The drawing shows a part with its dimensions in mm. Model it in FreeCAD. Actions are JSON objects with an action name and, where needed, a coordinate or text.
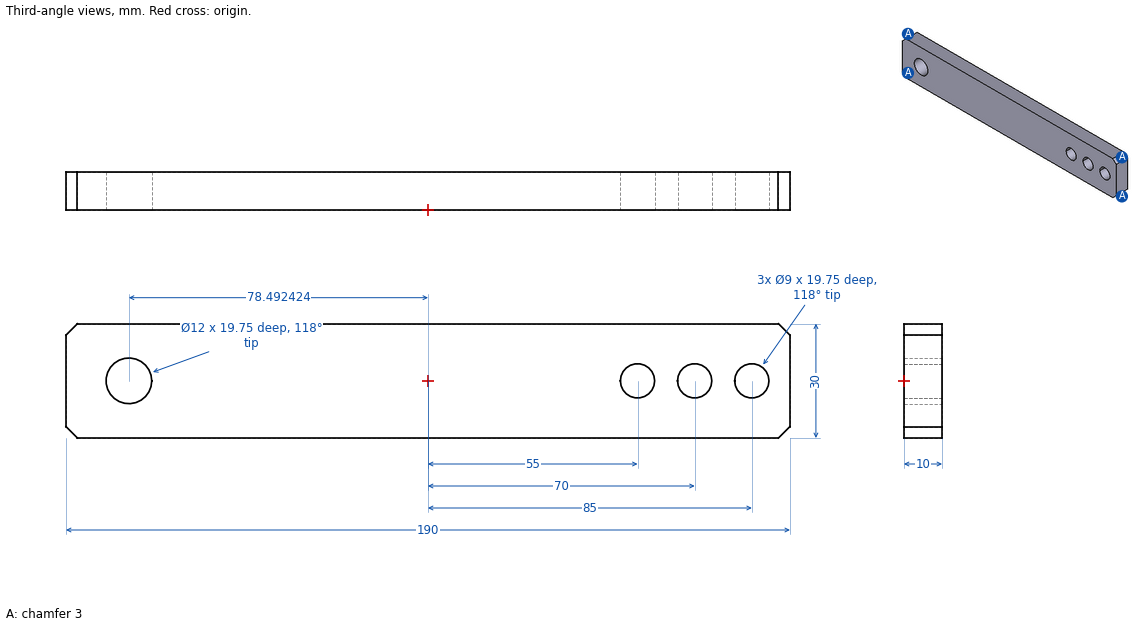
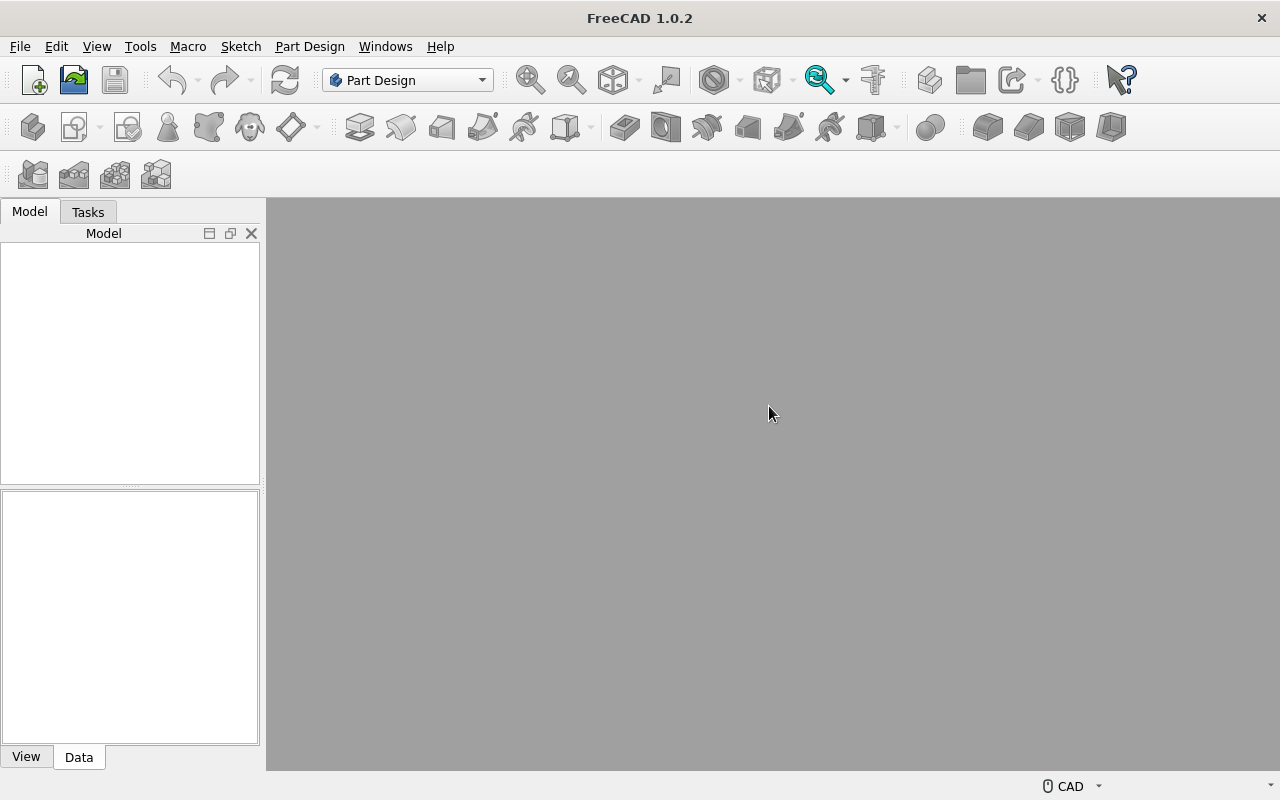
{"action": "key", "text": "ctrl+n"}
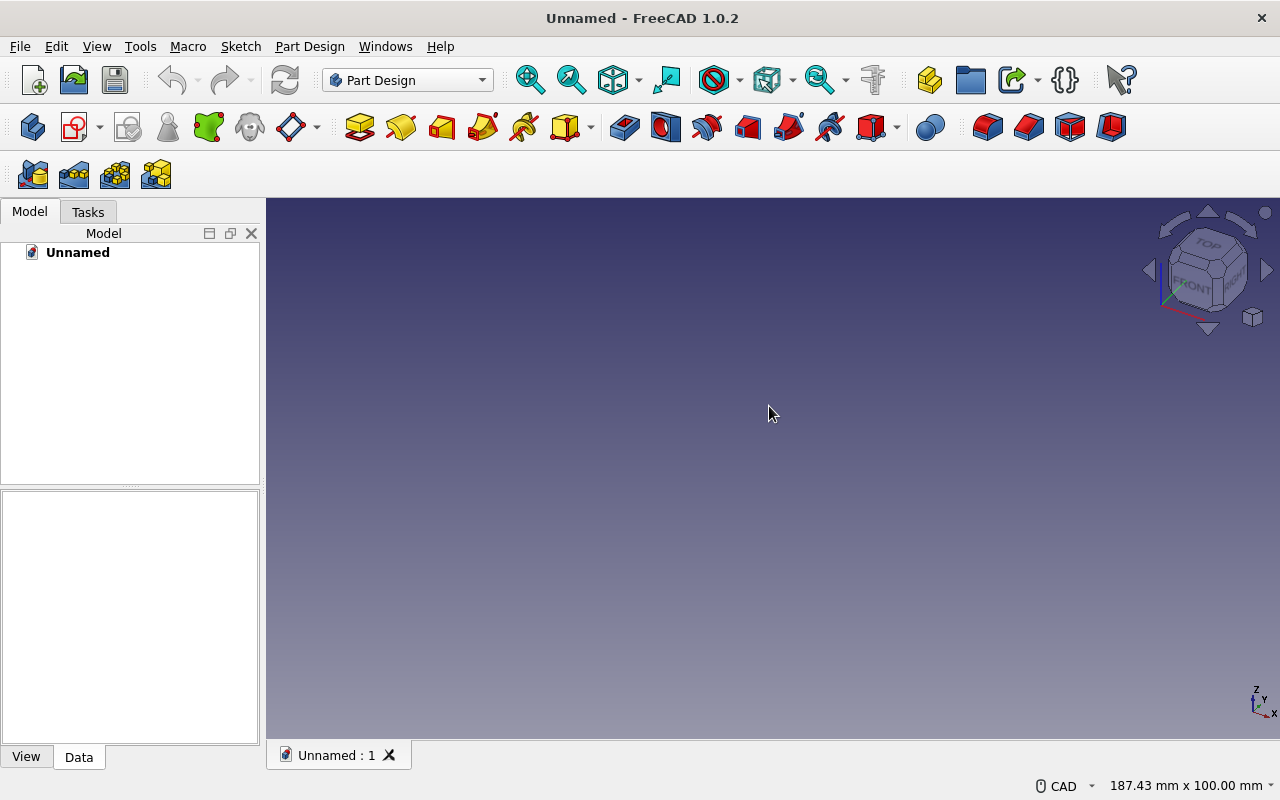
{"action": "left_click", "coordinate": [74, 128]}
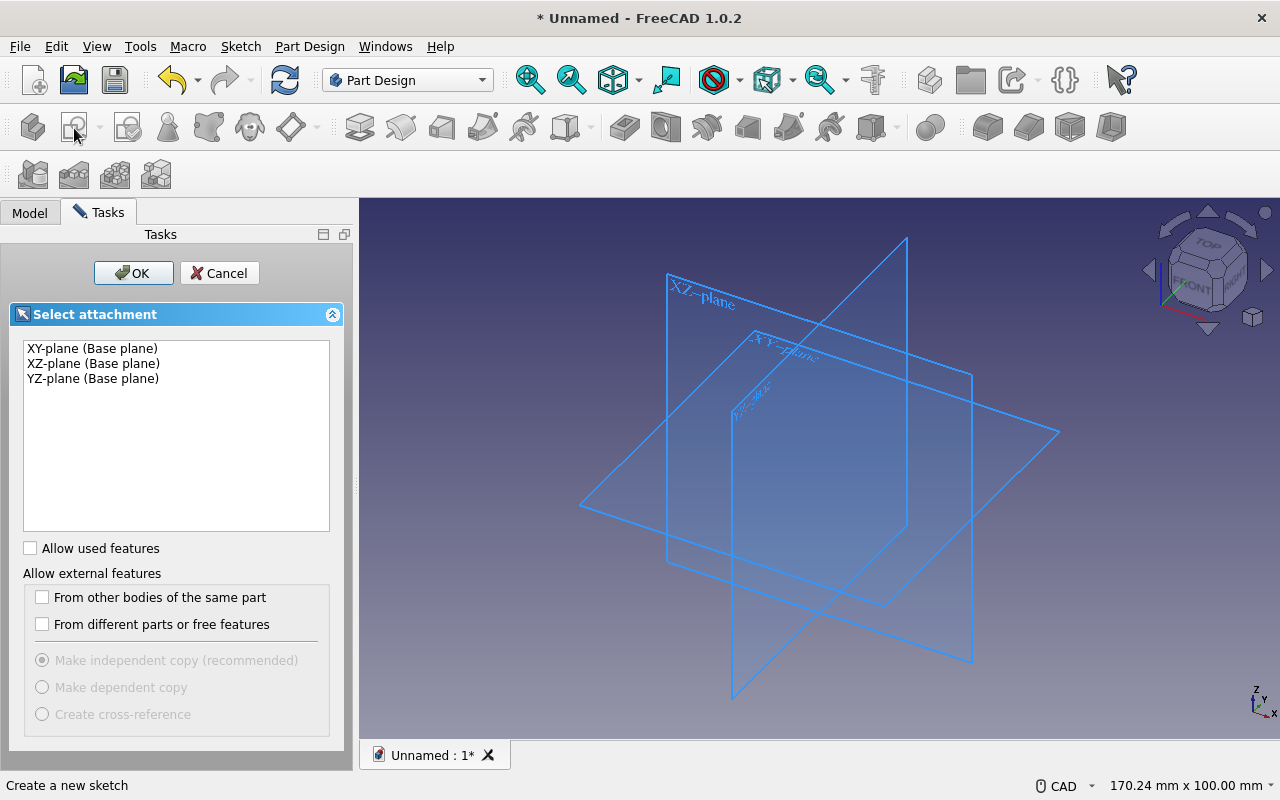
{"action": "left_click", "coordinate": [84, 364]}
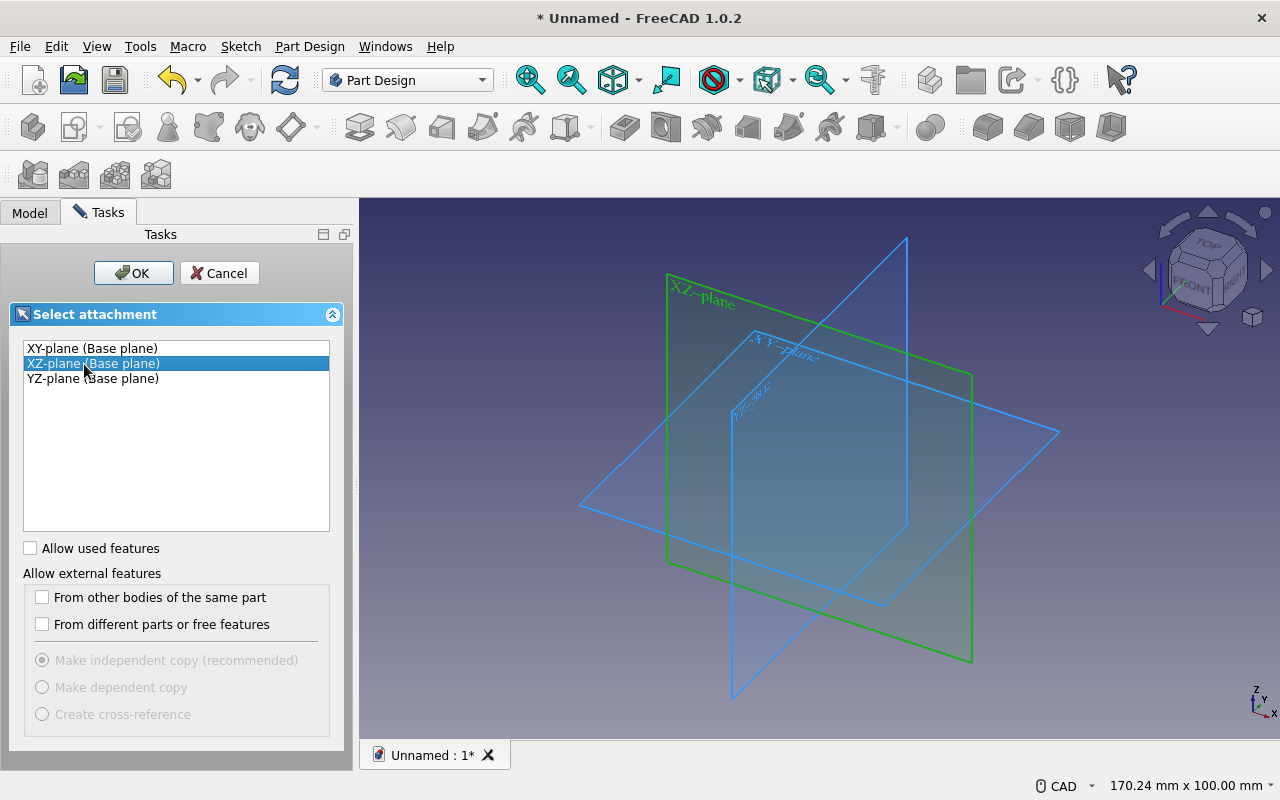
{"action": "left_click", "coordinate": [134, 273]}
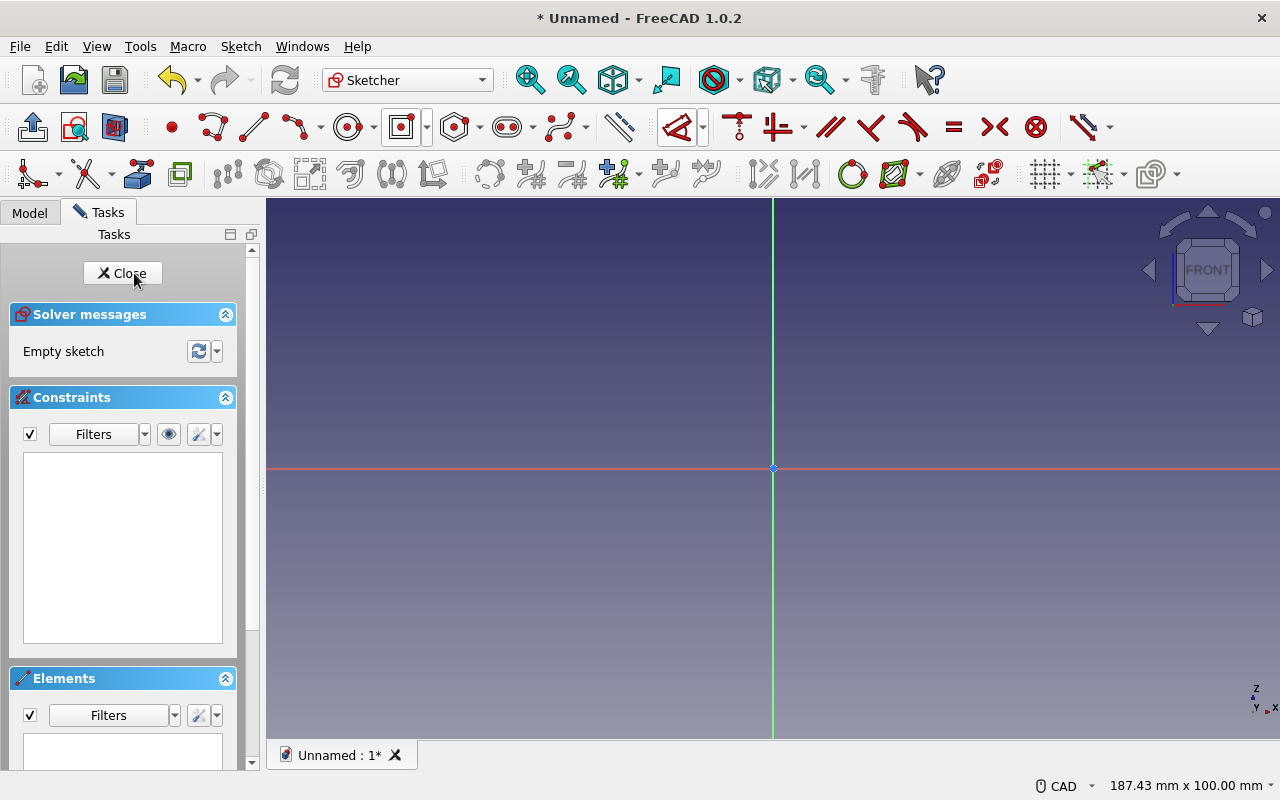
{"action": "scroll", "coordinate": [621, 468], "scroll_direction": "down", "scroll_amount": 3}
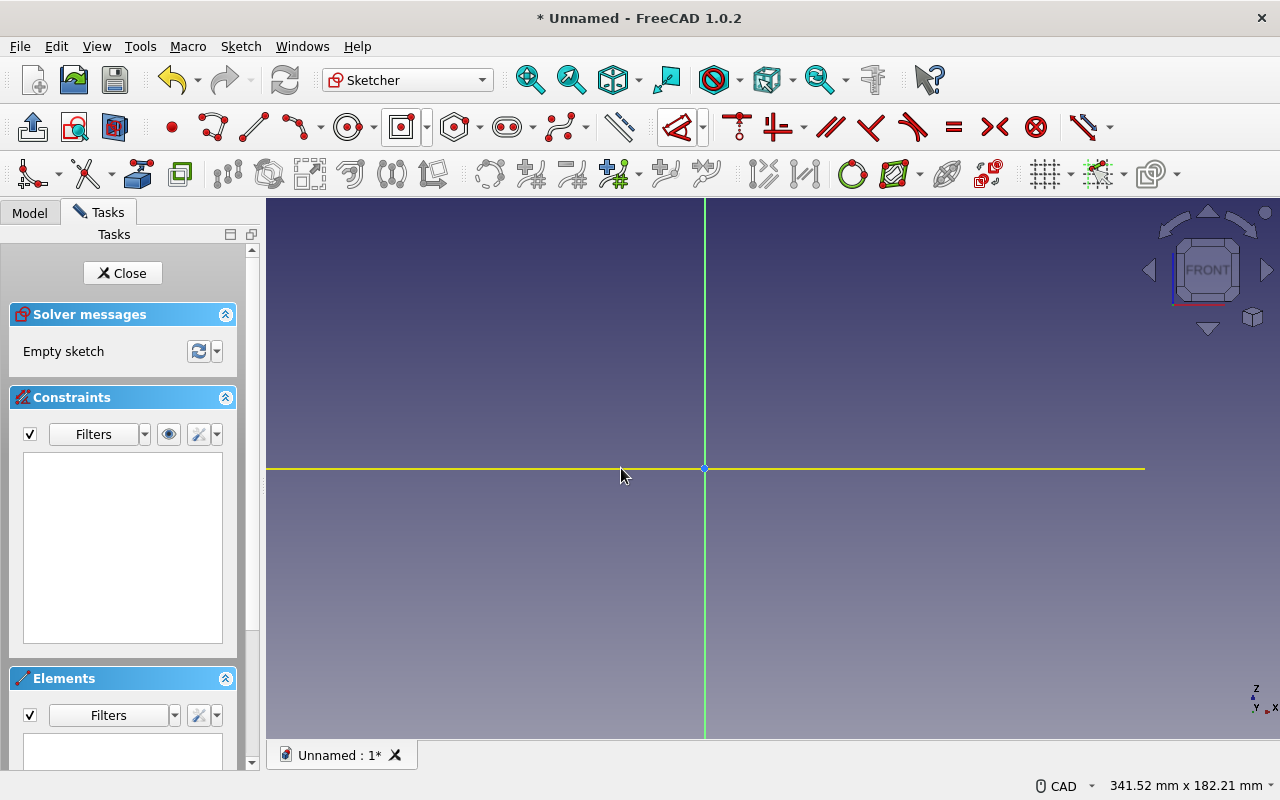
{"action": "left_click", "coordinate": [400, 128]}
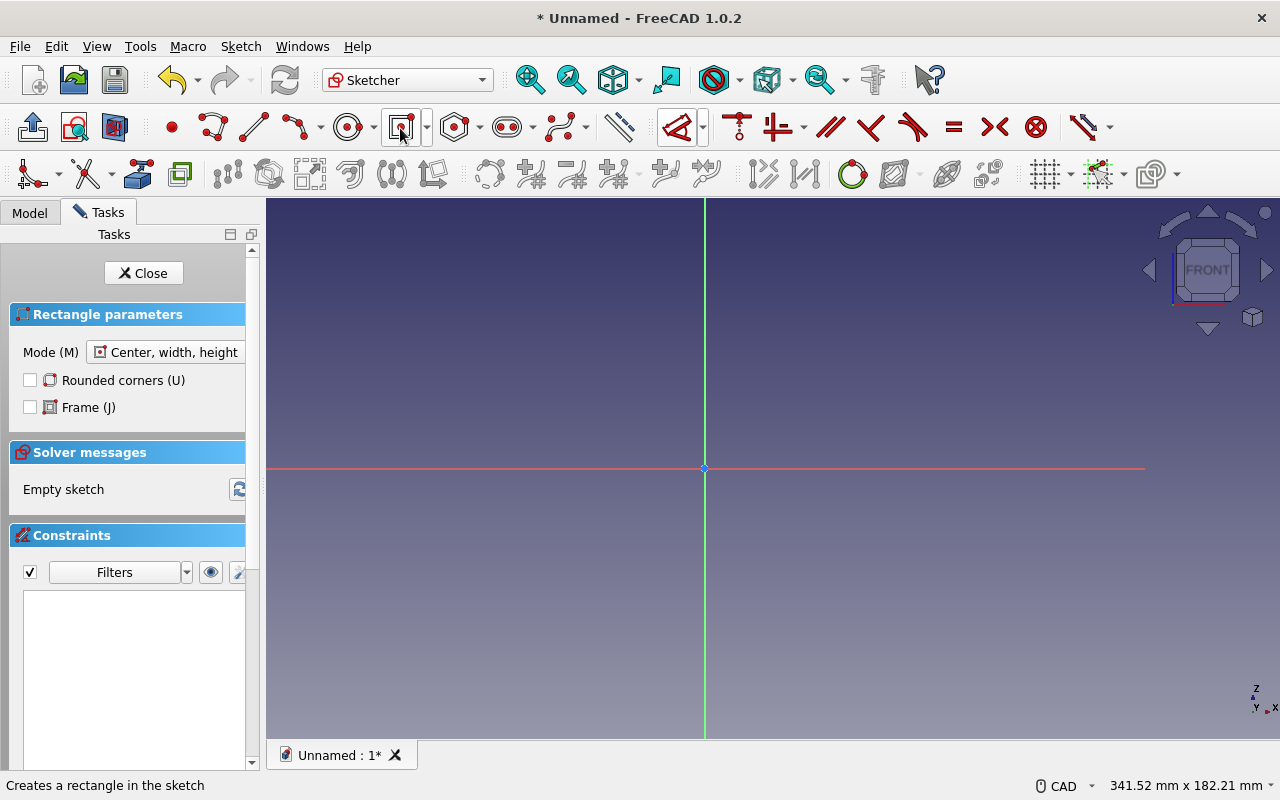
{"action": "left_click", "coordinate": [705, 468]}
{"action": "mouse_move", "coordinate": [987, 424]}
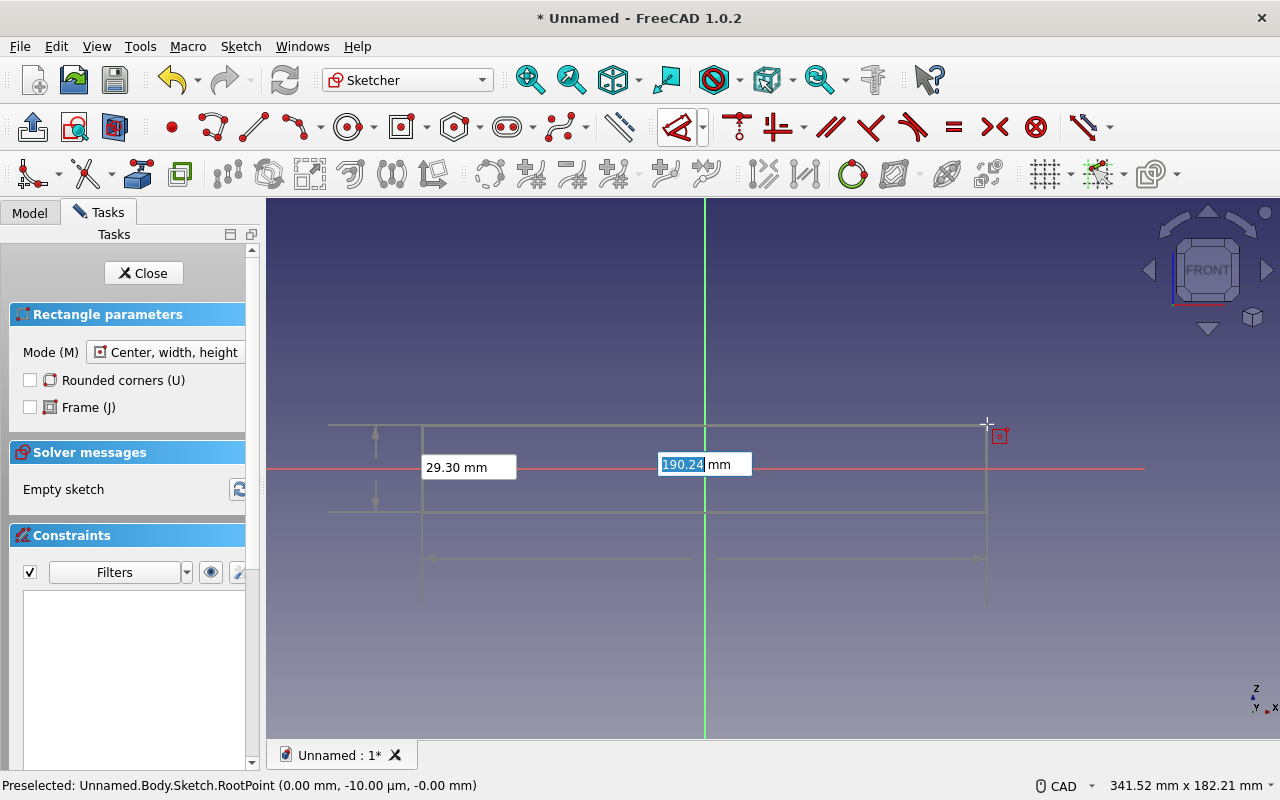
{"action": "type", "text": "190"}
{"action": "key", "text": "Tab"}
{"action": "type", "text": "30"}
{"action": "key", "text": "Return"}
{"action": "key", "text": "Escape"}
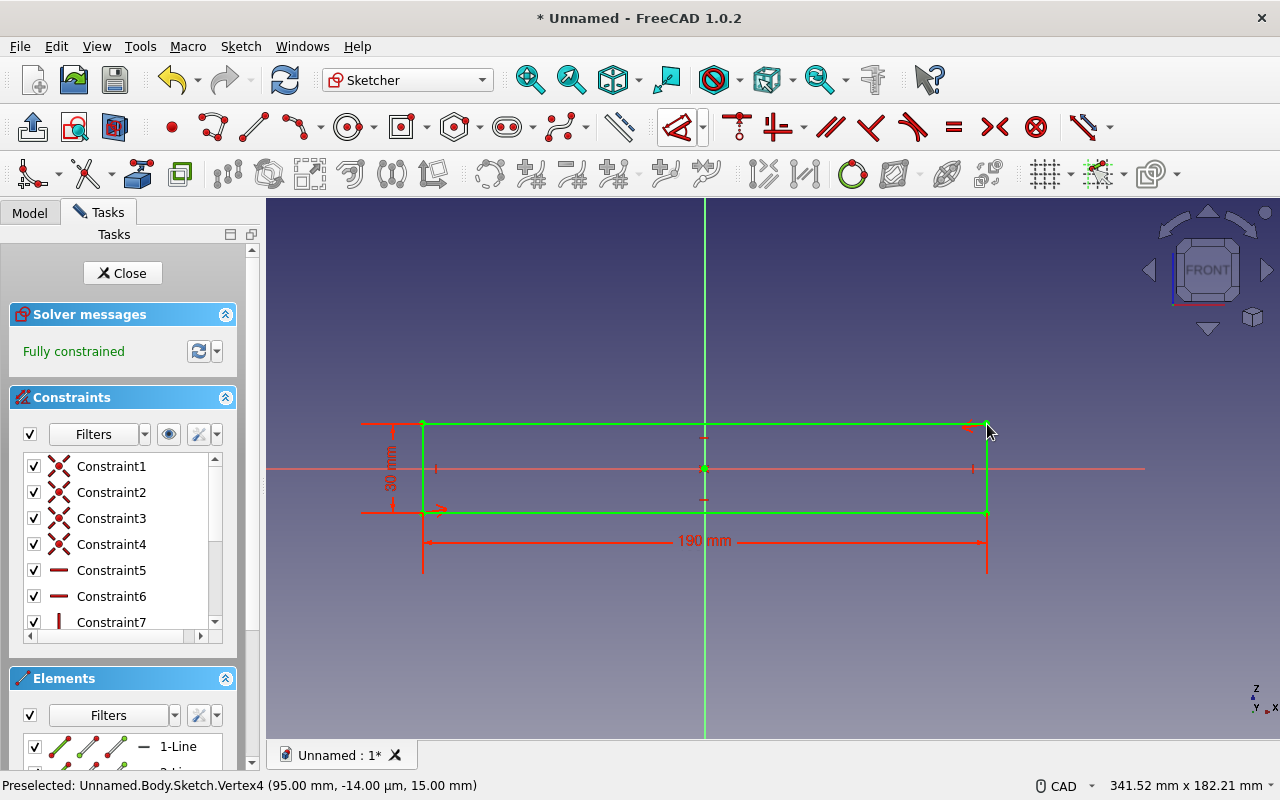
{"action": "left_click", "coordinate": [123, 273]}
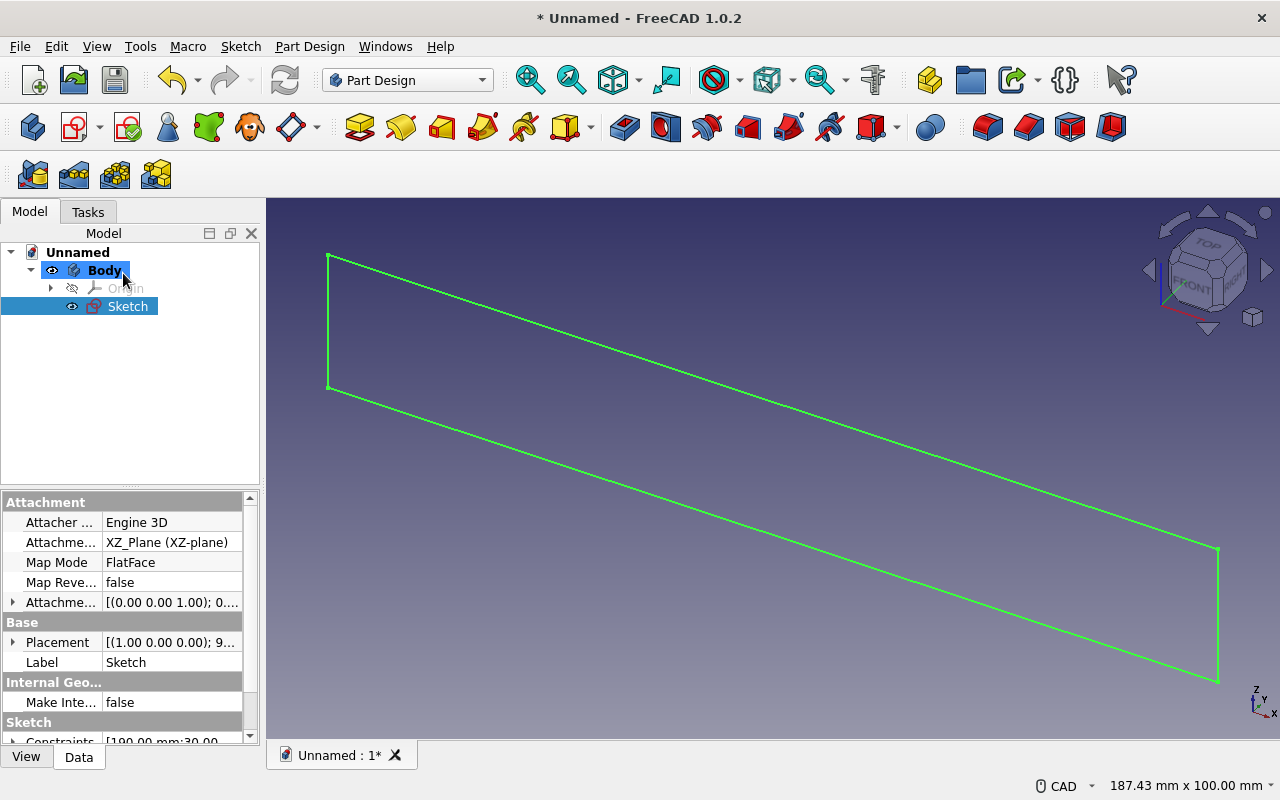
{"action": "left_click", "coordinate": [360, 128]}